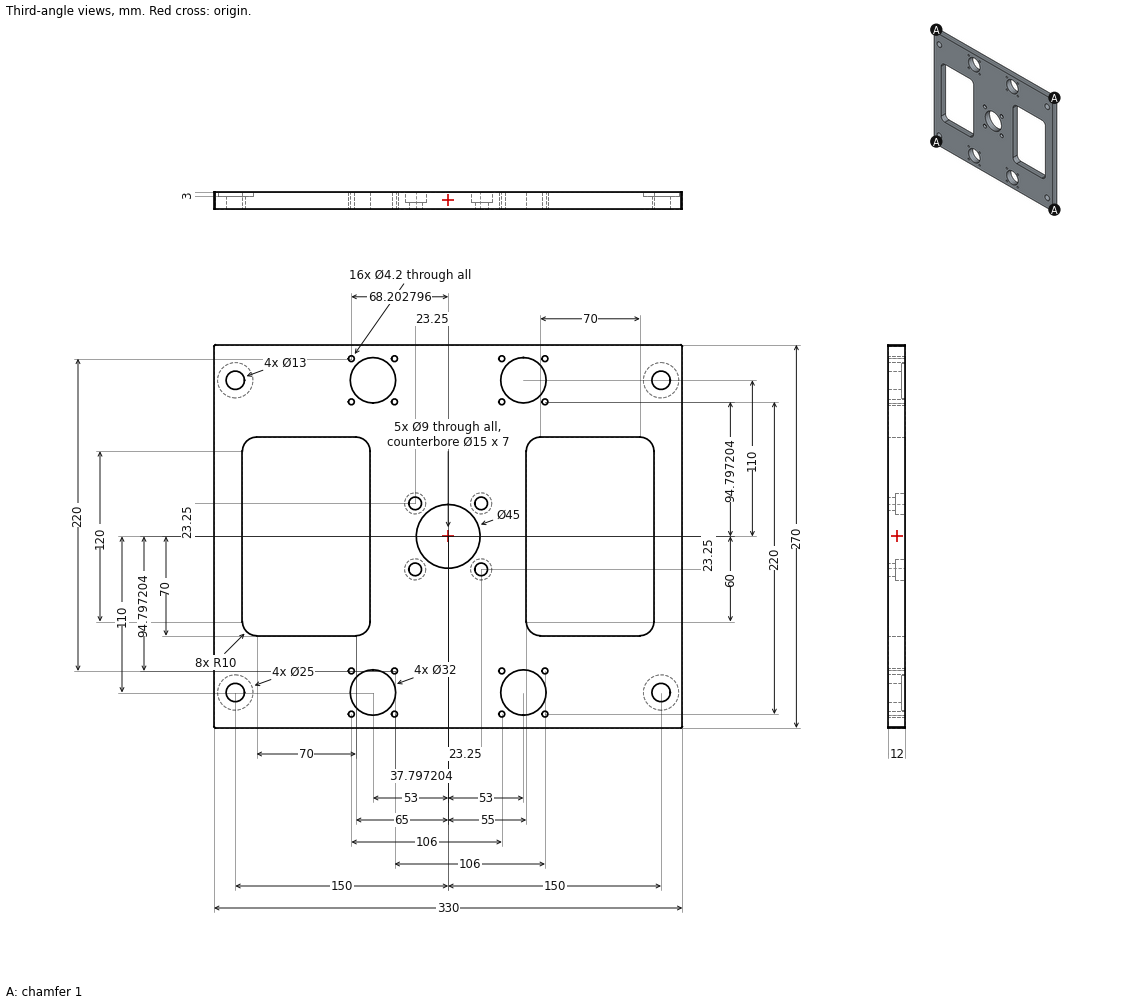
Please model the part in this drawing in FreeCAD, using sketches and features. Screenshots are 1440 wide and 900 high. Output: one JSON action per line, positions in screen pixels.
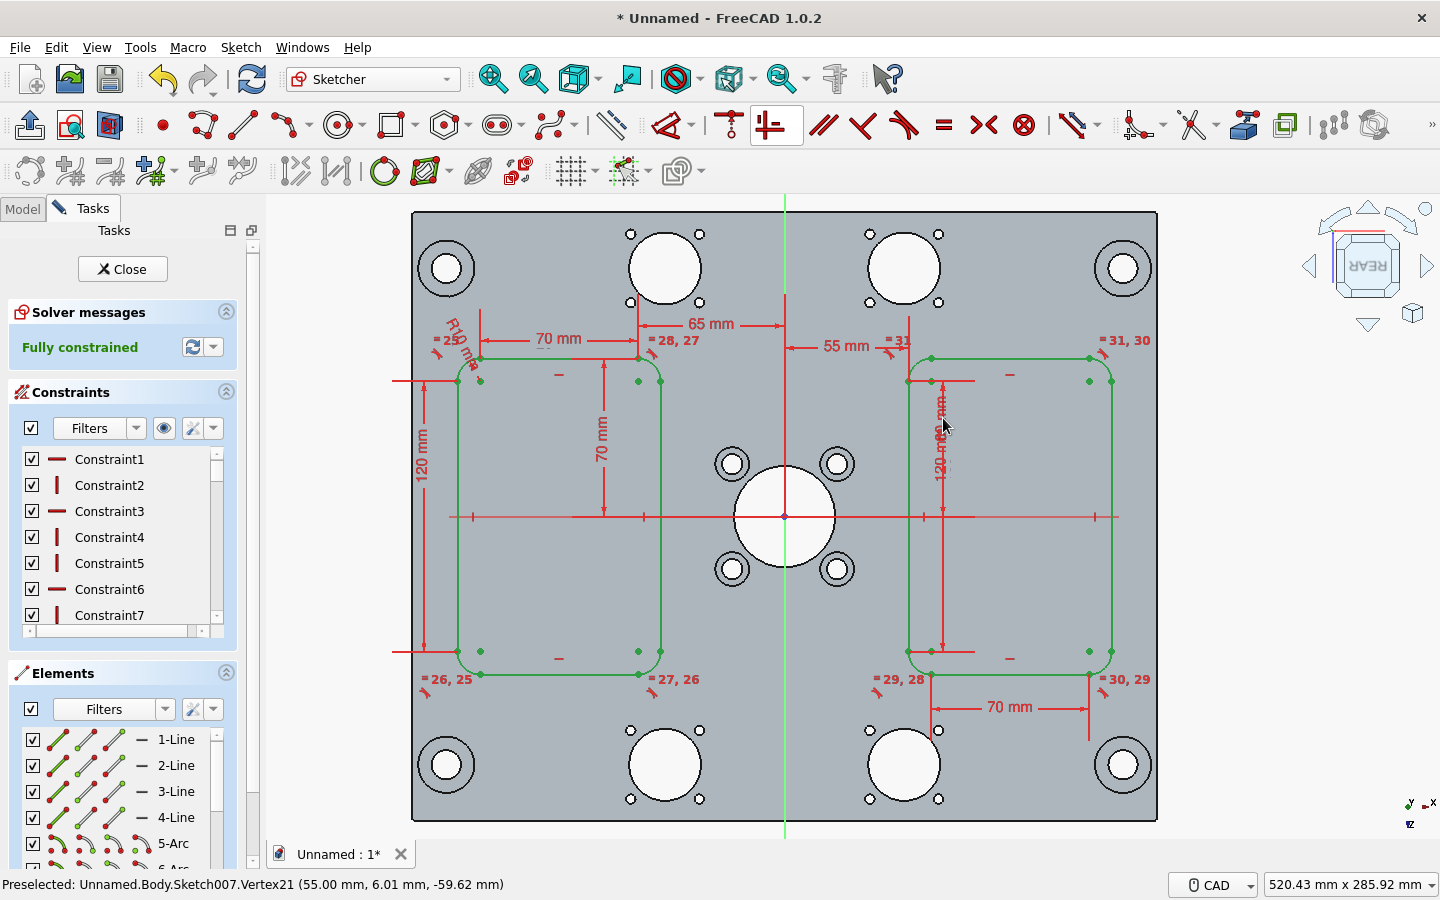
{"action": "left_click", "coordinate": [123, 269]}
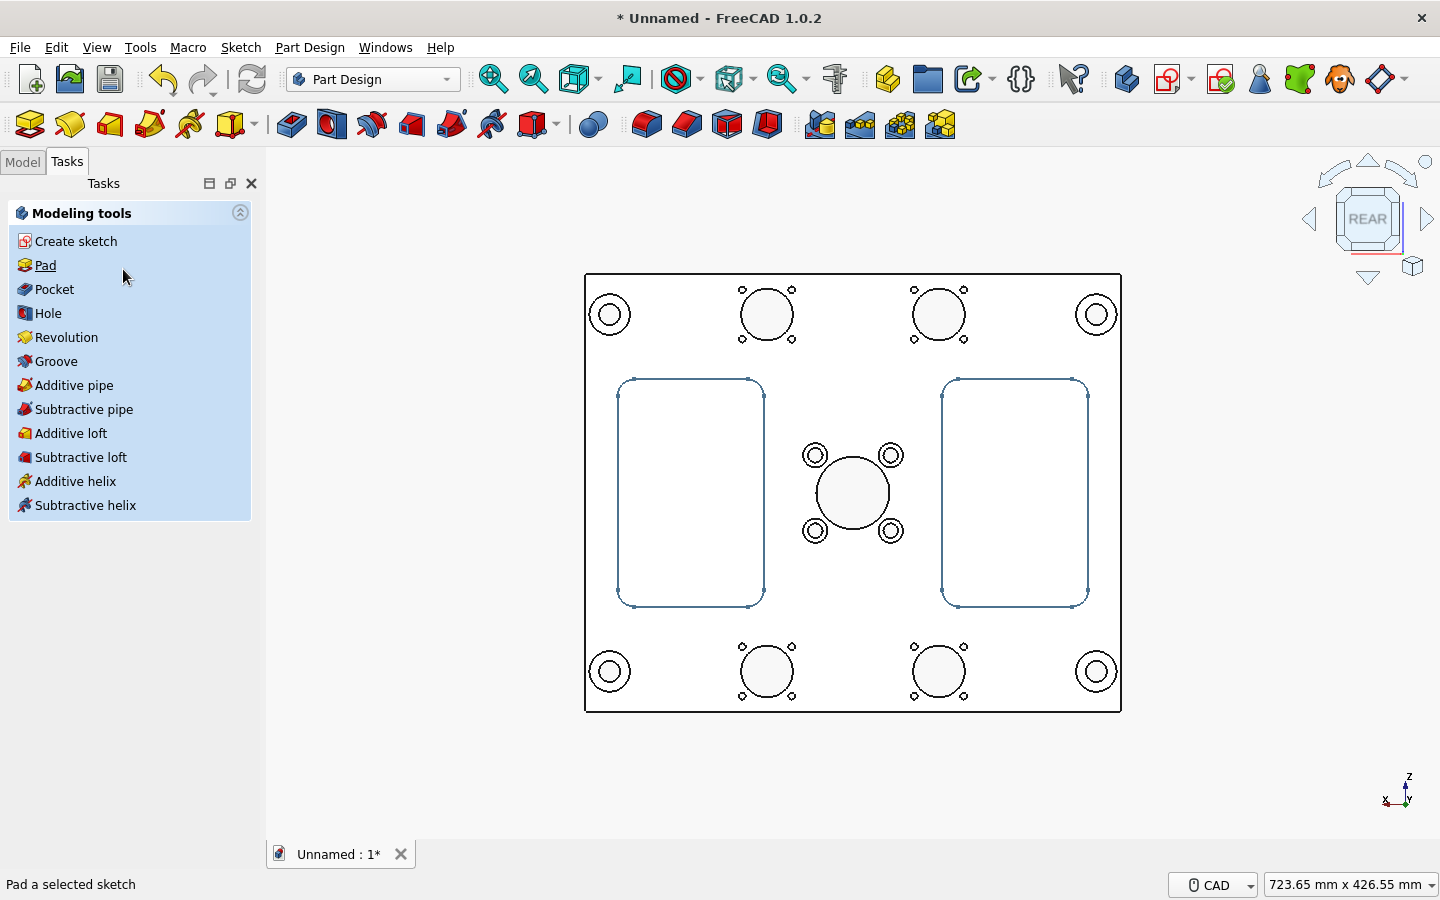
{"action": "left_click", "coordinate": [292, 124]}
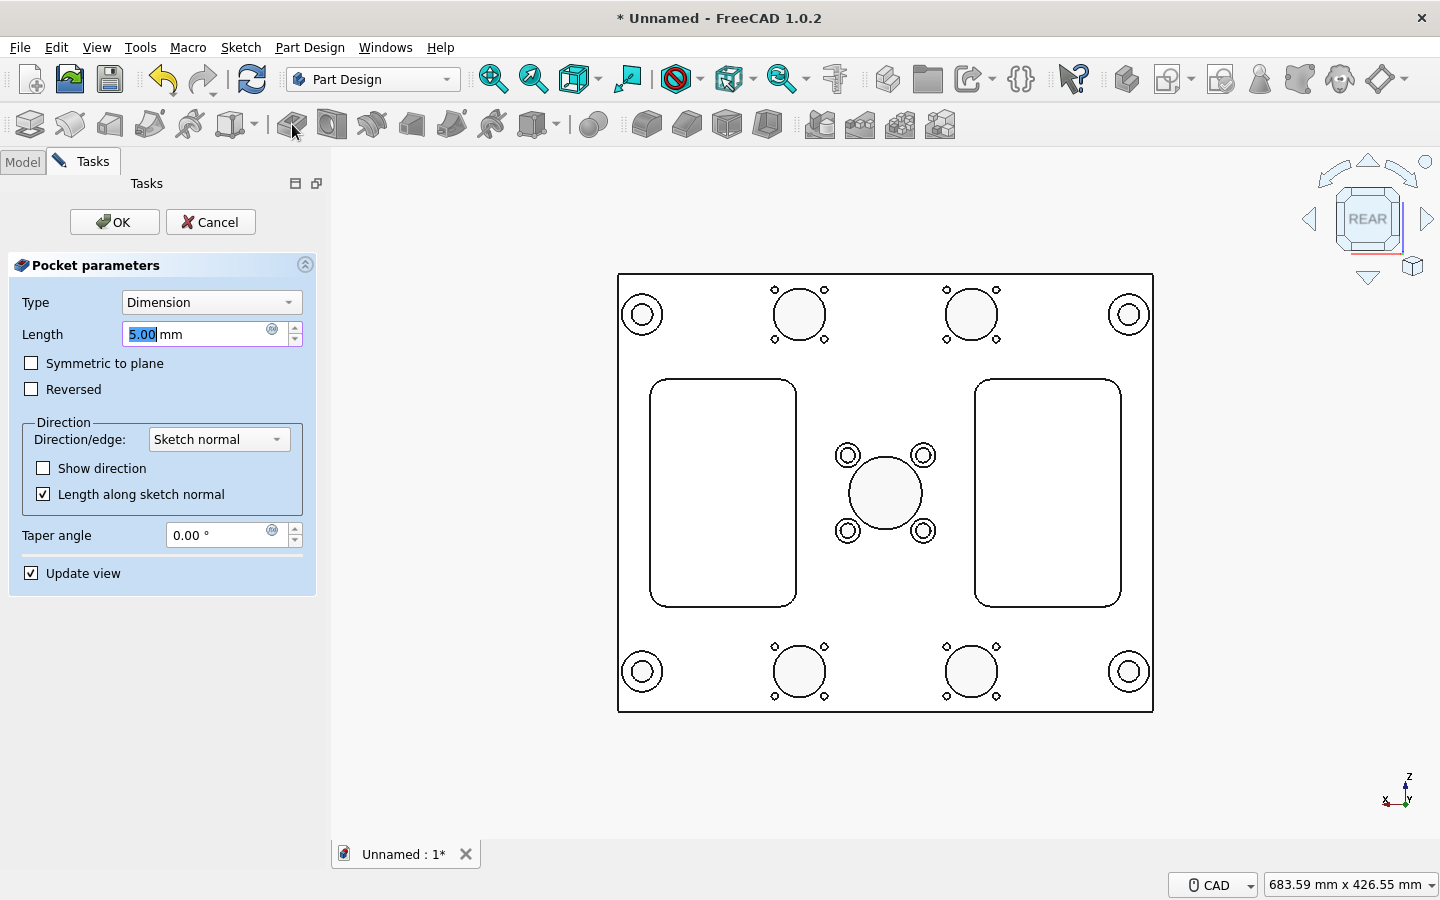
{"action": "left_click", "coordinate": [212, 302]}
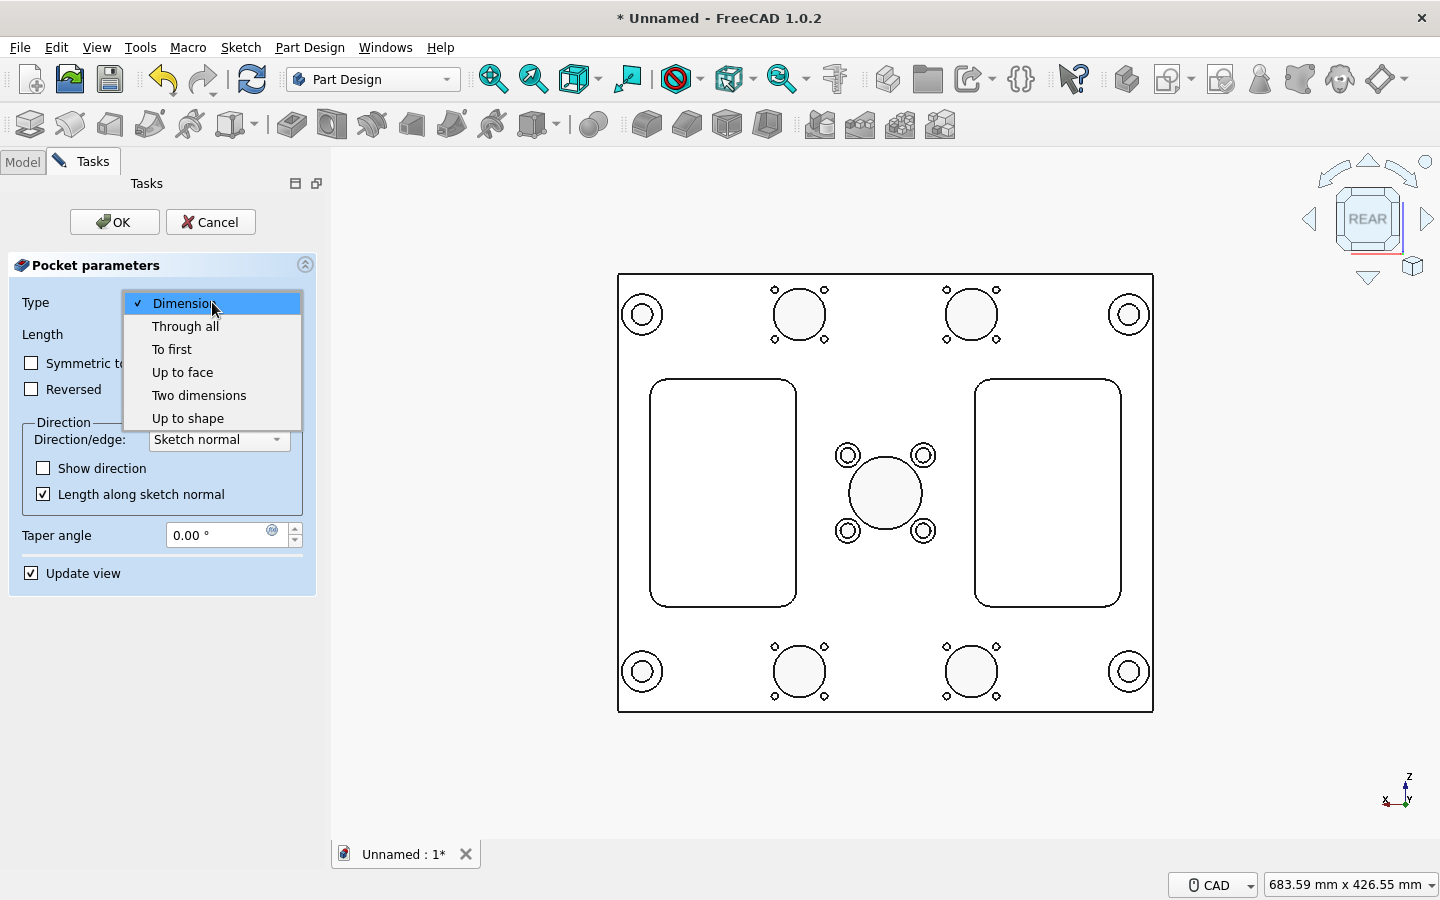
{"action": "left_click", "coordinate": [212, 326]}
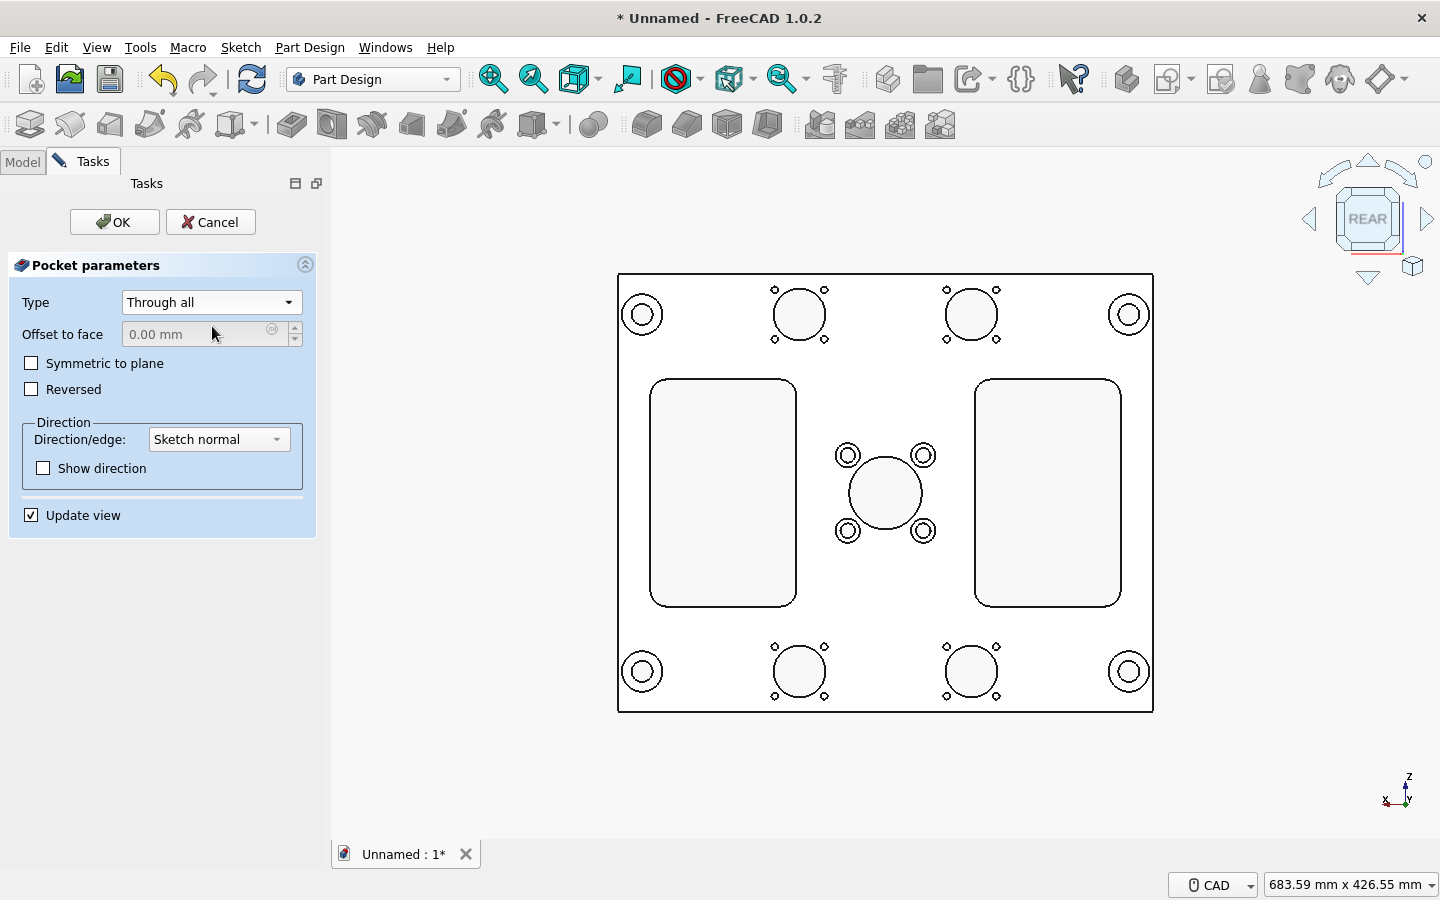
{"action": "left_click", "coordinate": [115, 222]}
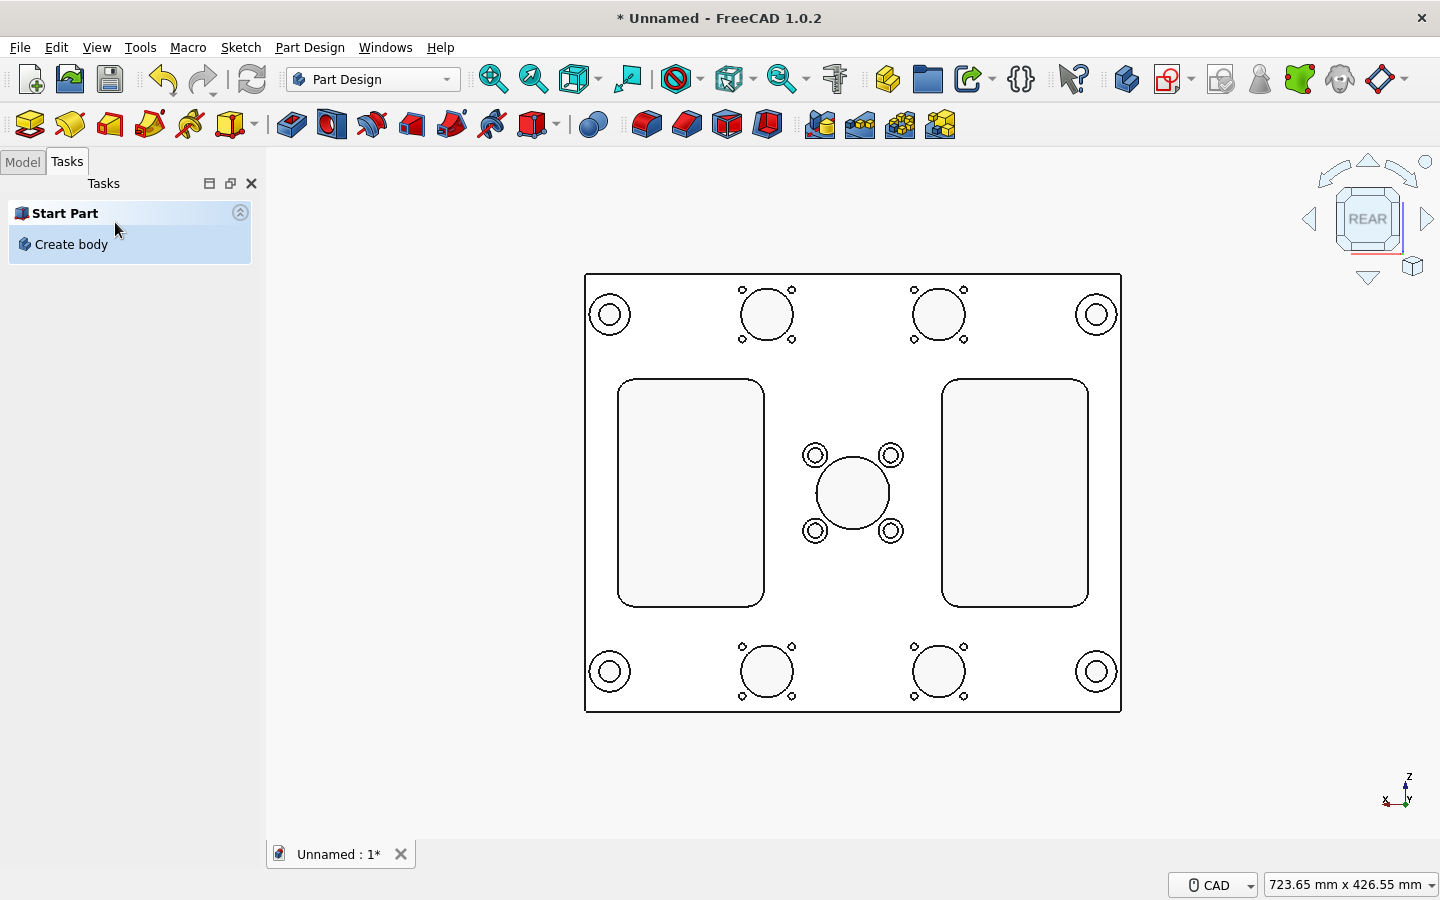
{"action": "key", "text": "0"}